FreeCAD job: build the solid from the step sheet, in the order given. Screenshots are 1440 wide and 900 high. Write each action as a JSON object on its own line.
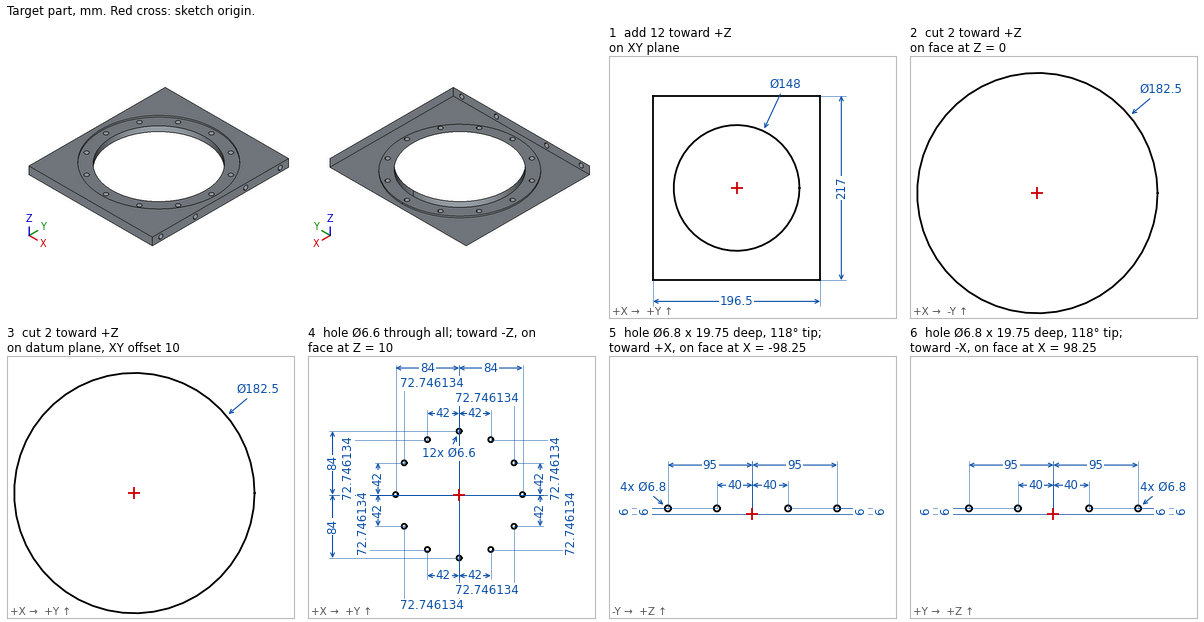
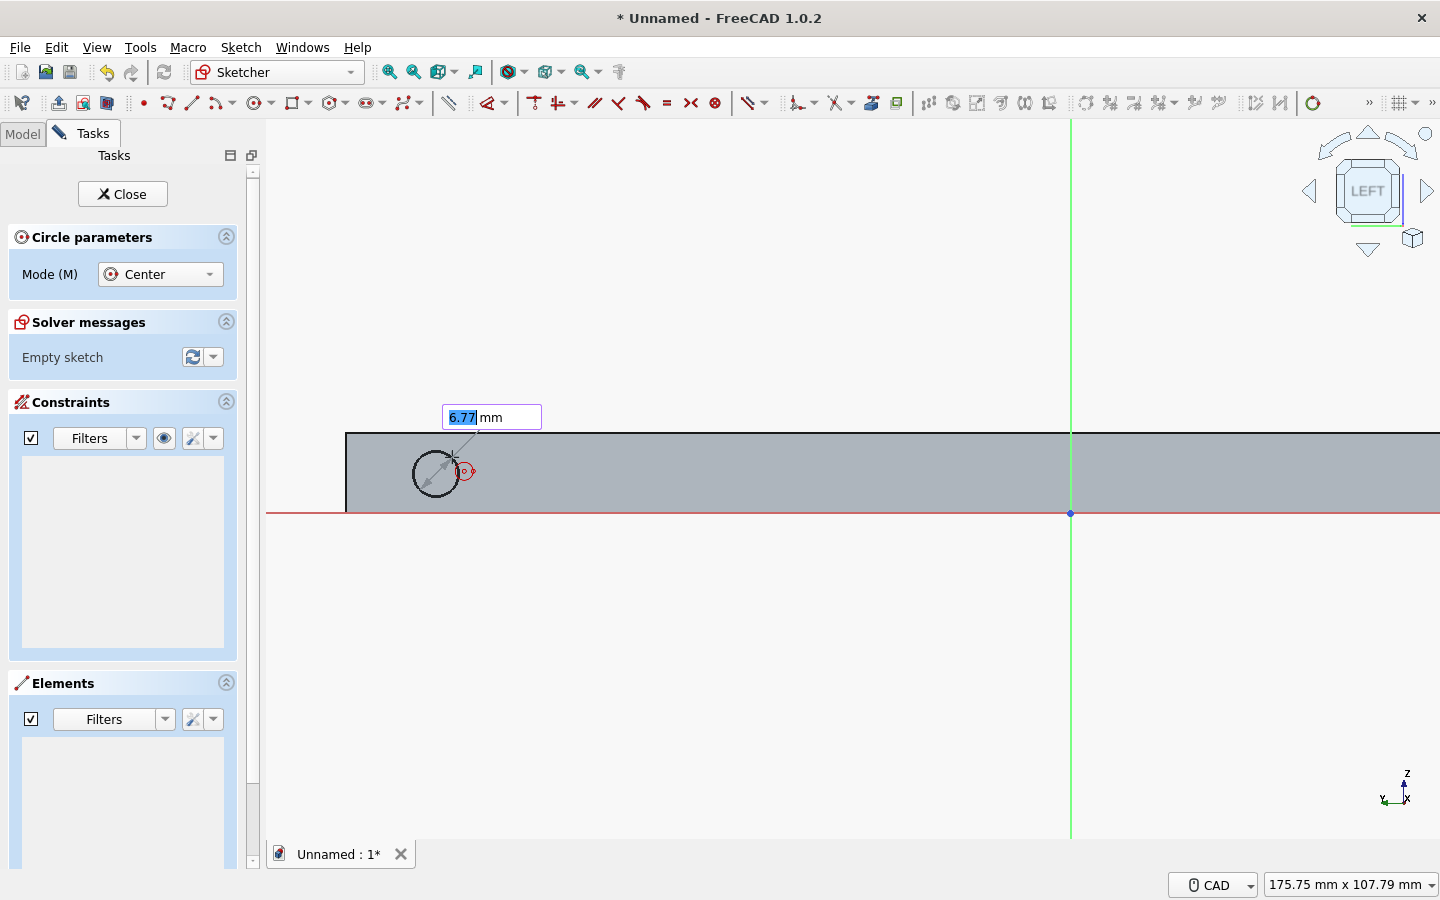
{"action": "type", "text": "6.8"}
{"action": "key", "text": "Return"}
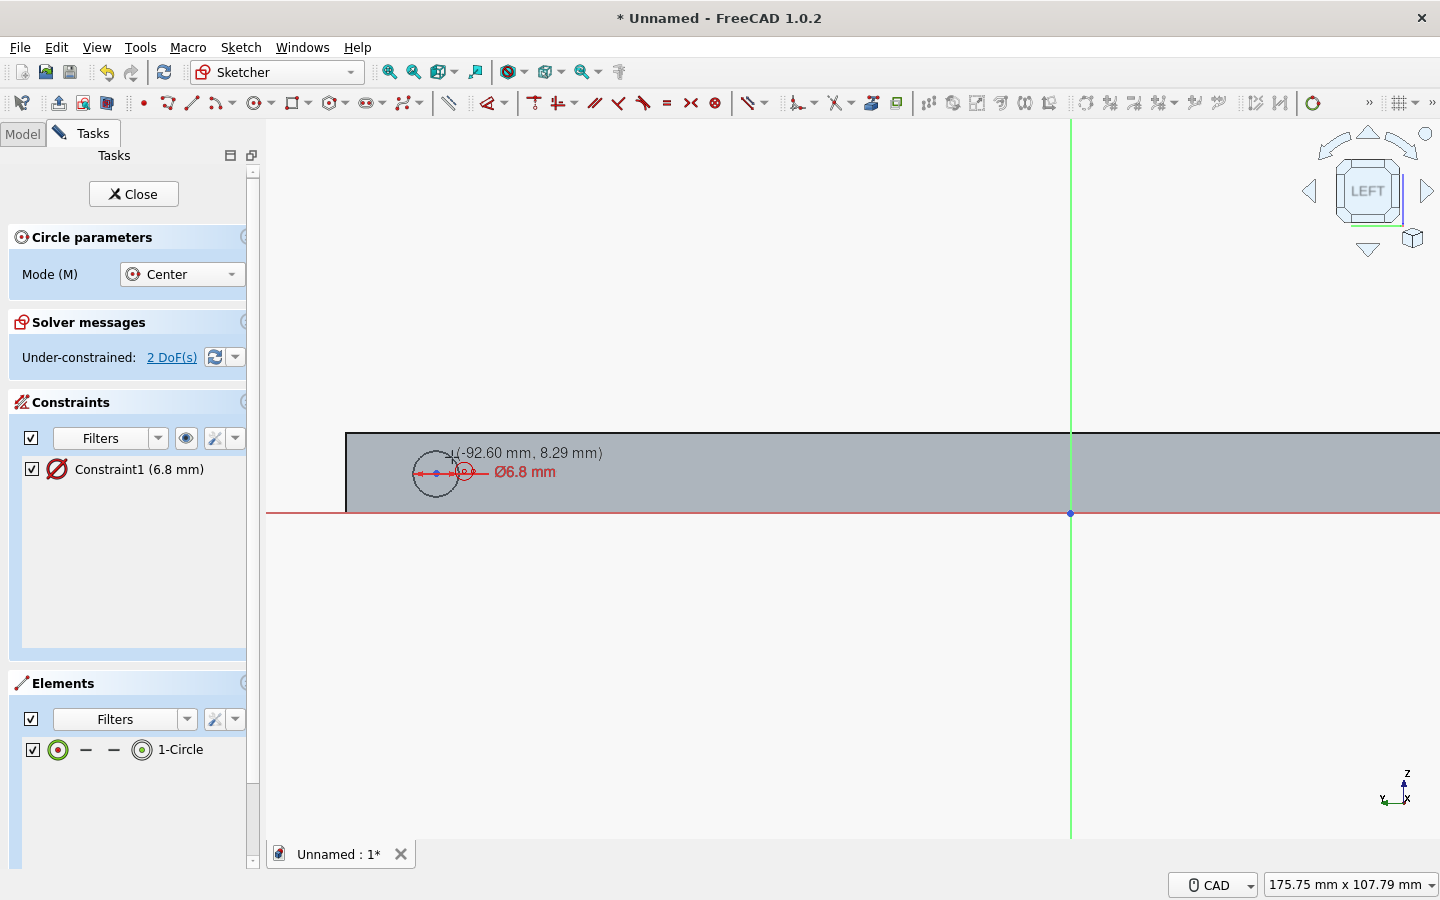
{"action": "left_click", "coordinate": [803, 473]}
{"action": "mouse_move", "coordinate": [819, 457]}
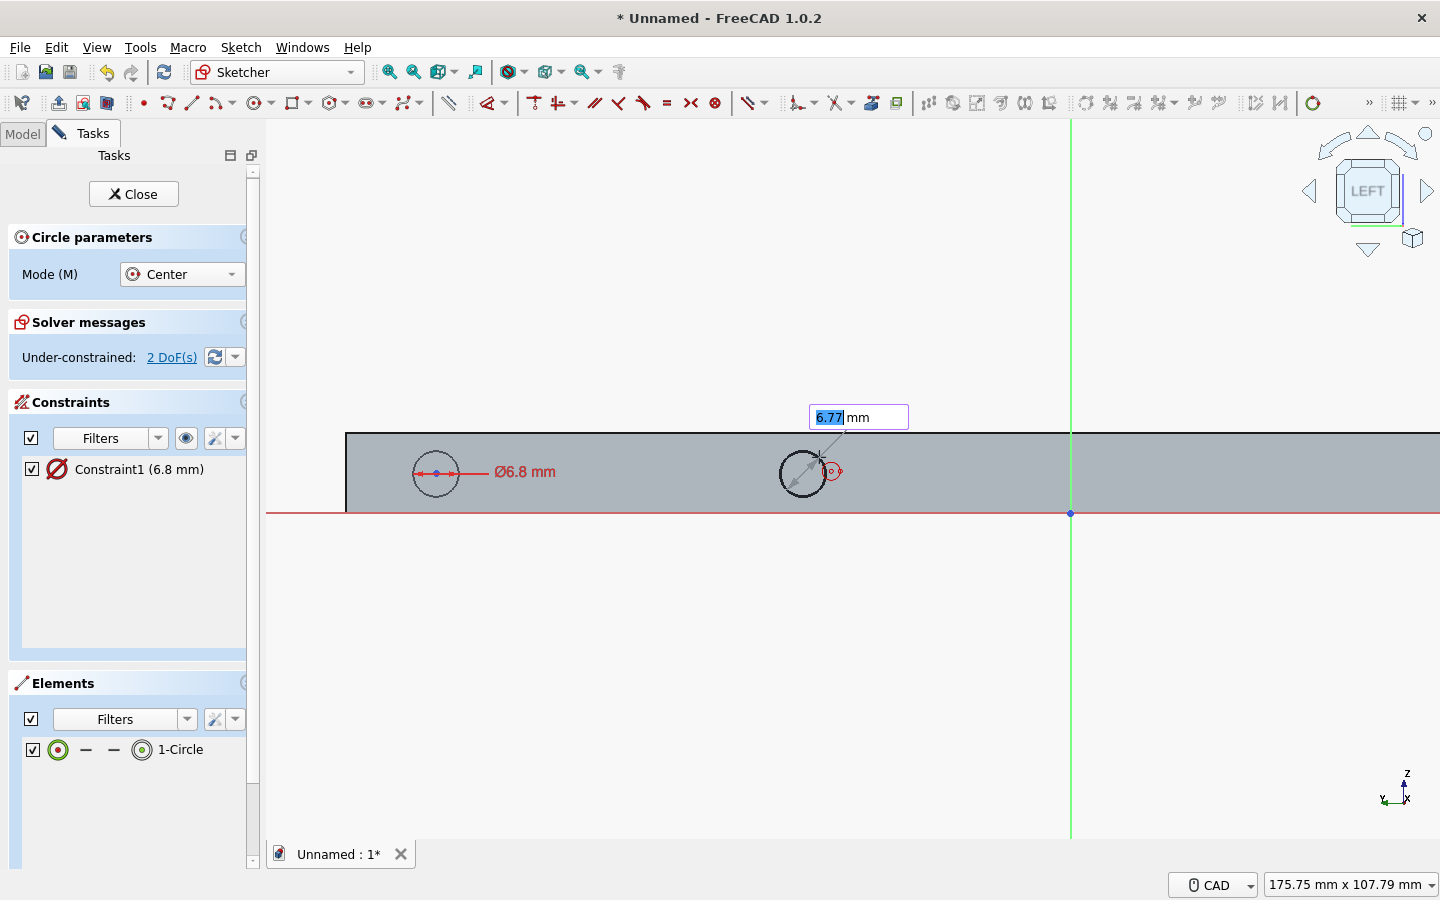
{"action": "type", "text": "6.8"}
{"action": "key", "text": "Return"}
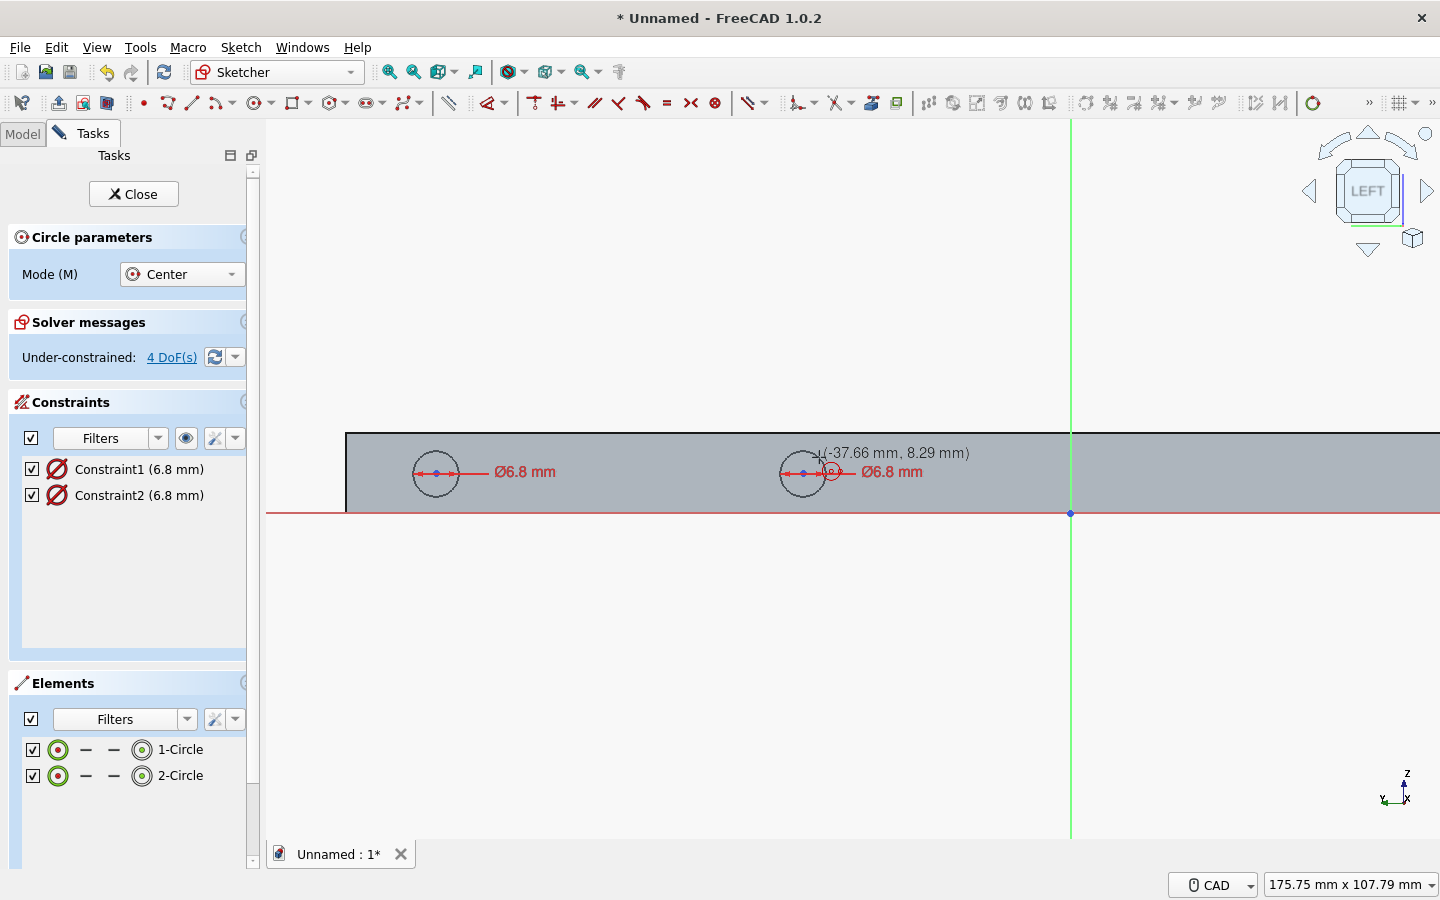
{"action": "scroll", "coordinate": [437, 475], "scroll_direction": "down", "scroll_amount": 3}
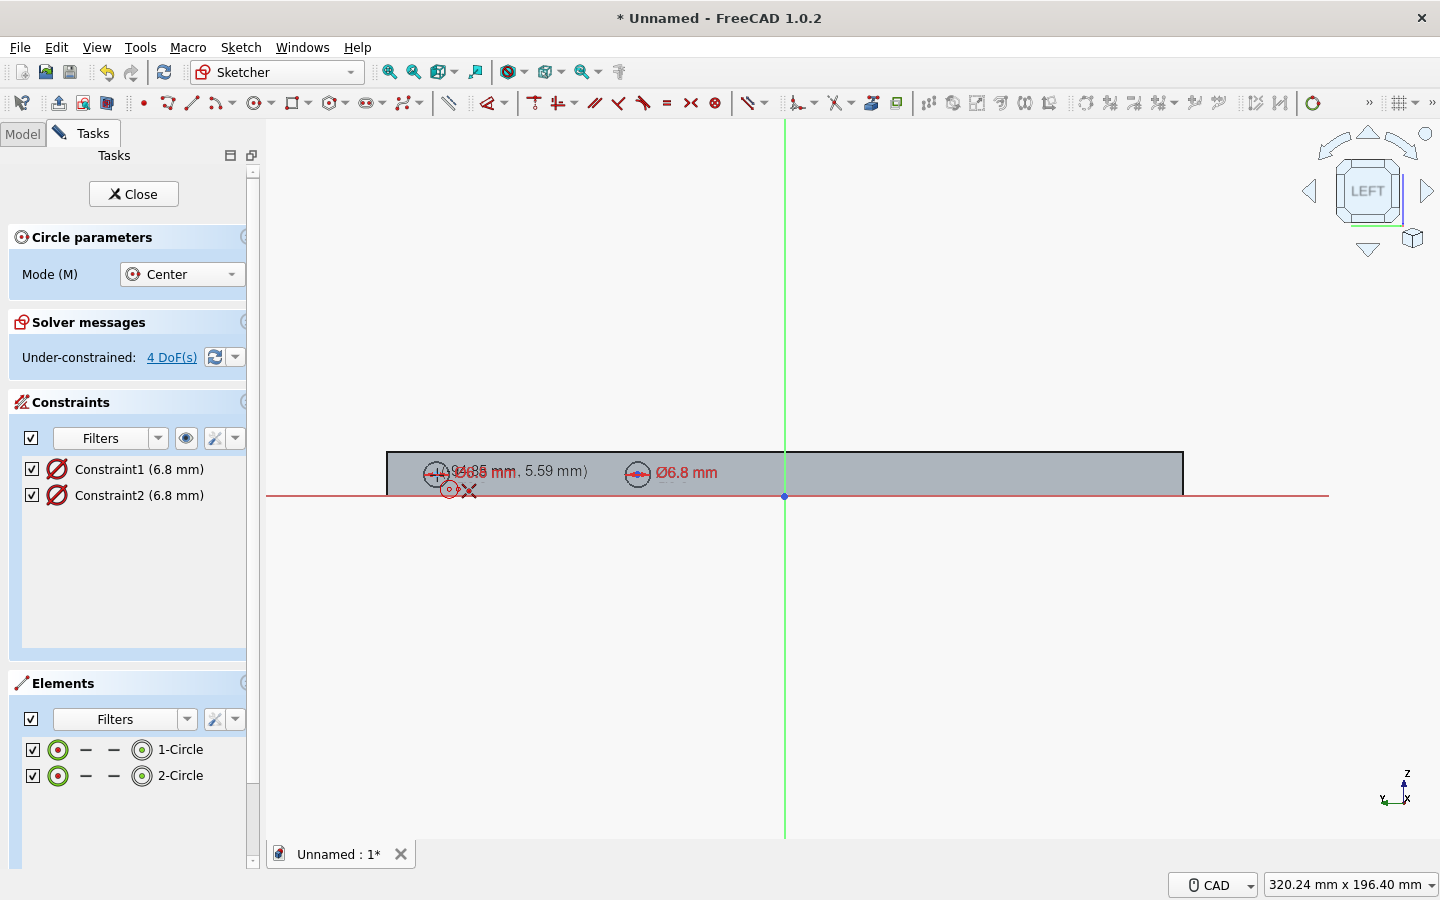
{"action": "scroll", "coordinate": [931, 474], "scroll_direction": "up", "scroll_amount": 3}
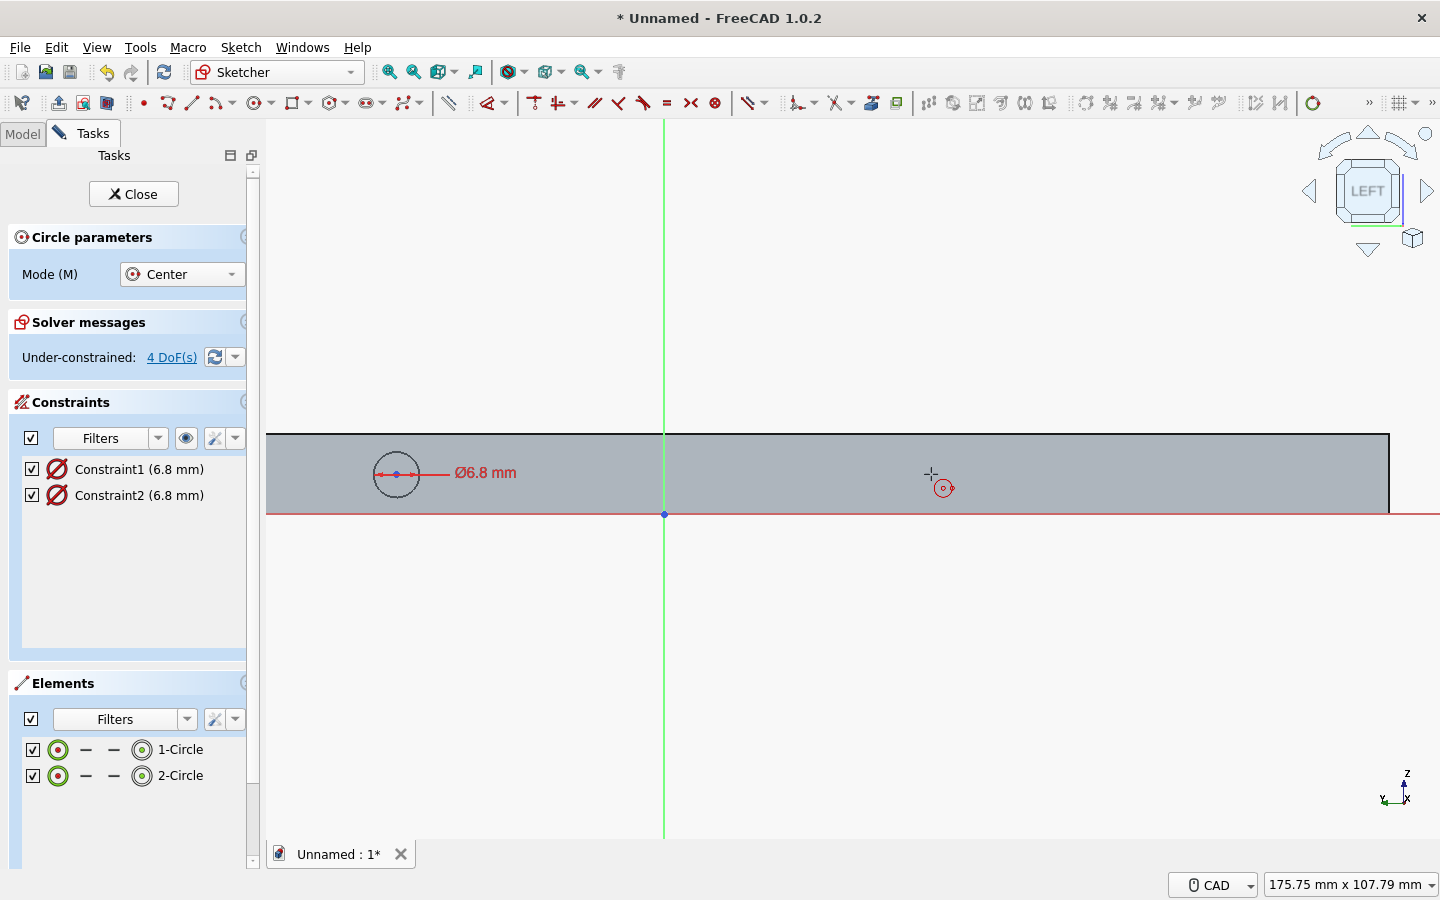
{"action": "left_click", "coordinate": [931, 474]}
{"action": "mouse_move", "coordinate": [947, 458]}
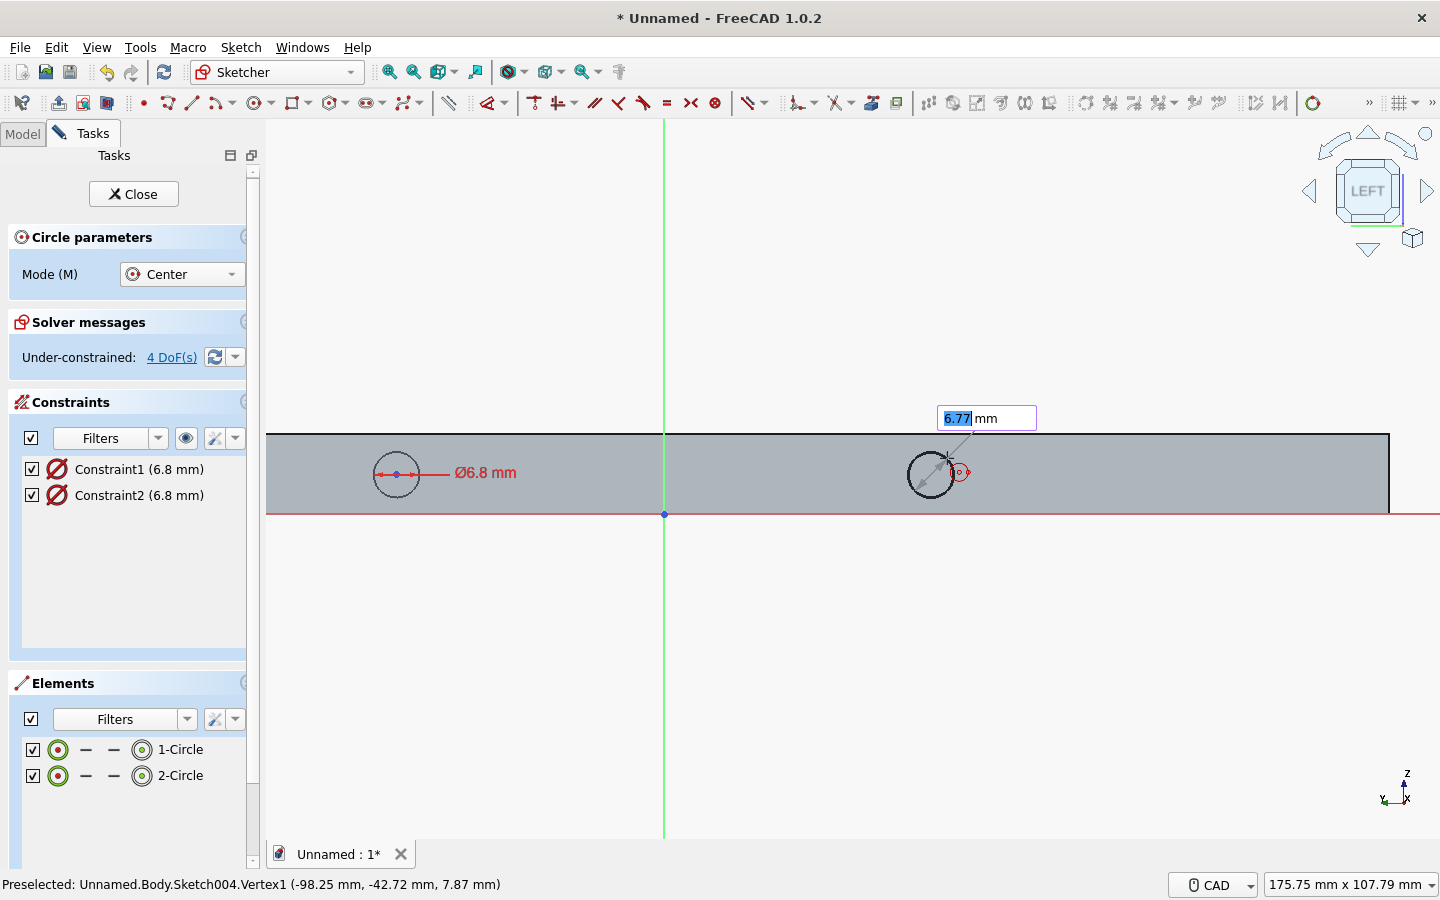
{"action": "type", "text": "6.8"}
{"action": "key", "text": "Return"}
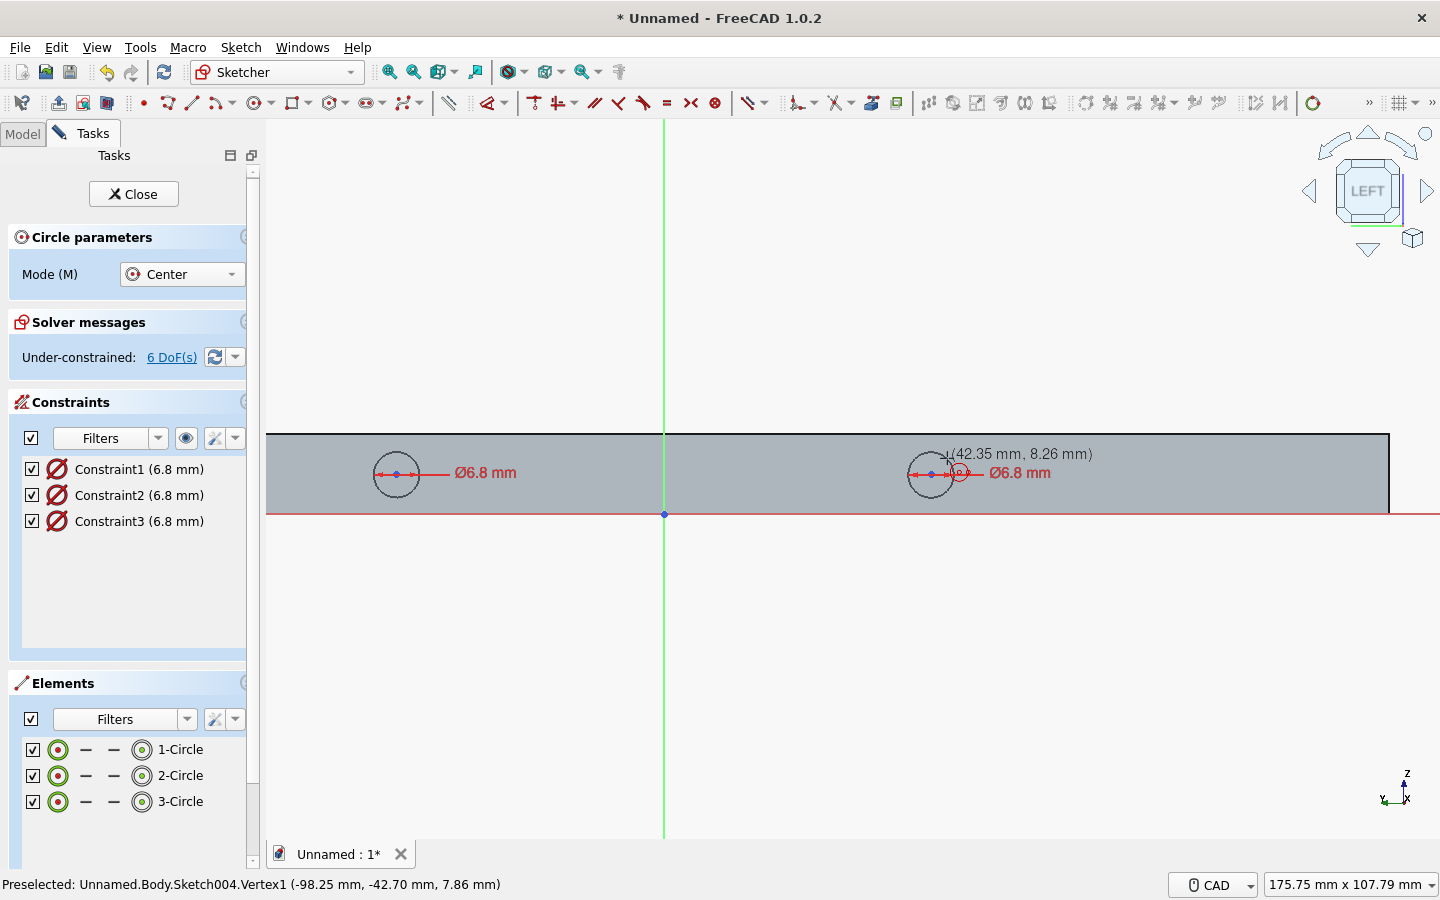
{"action": "scroll", "coordinate": [931, 474], "scroll_direction": "down", "scroll_amount": 3}